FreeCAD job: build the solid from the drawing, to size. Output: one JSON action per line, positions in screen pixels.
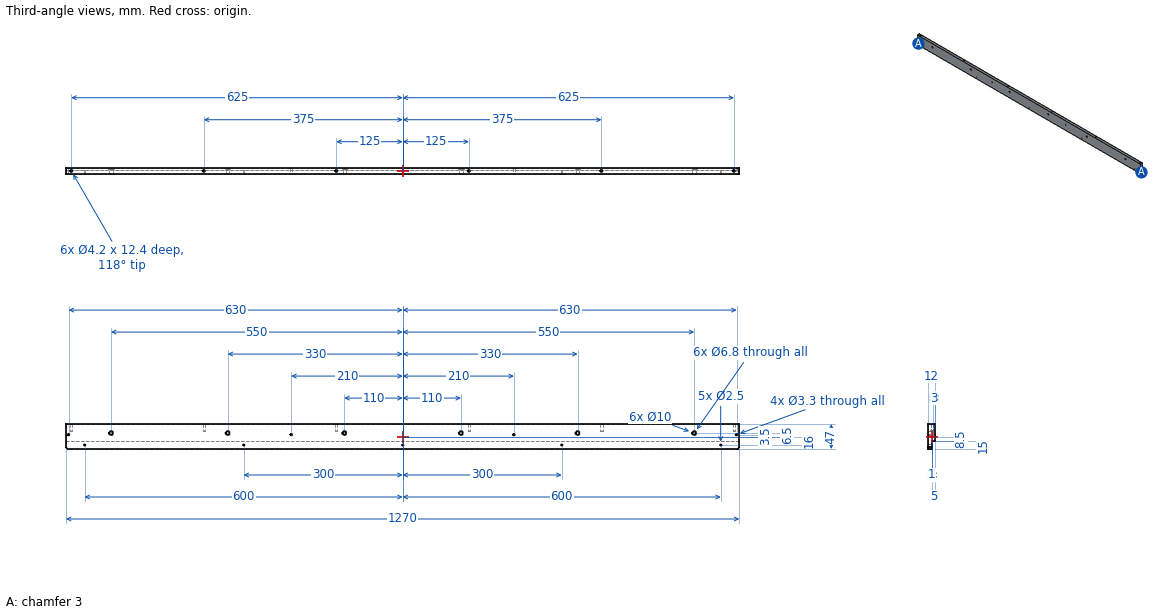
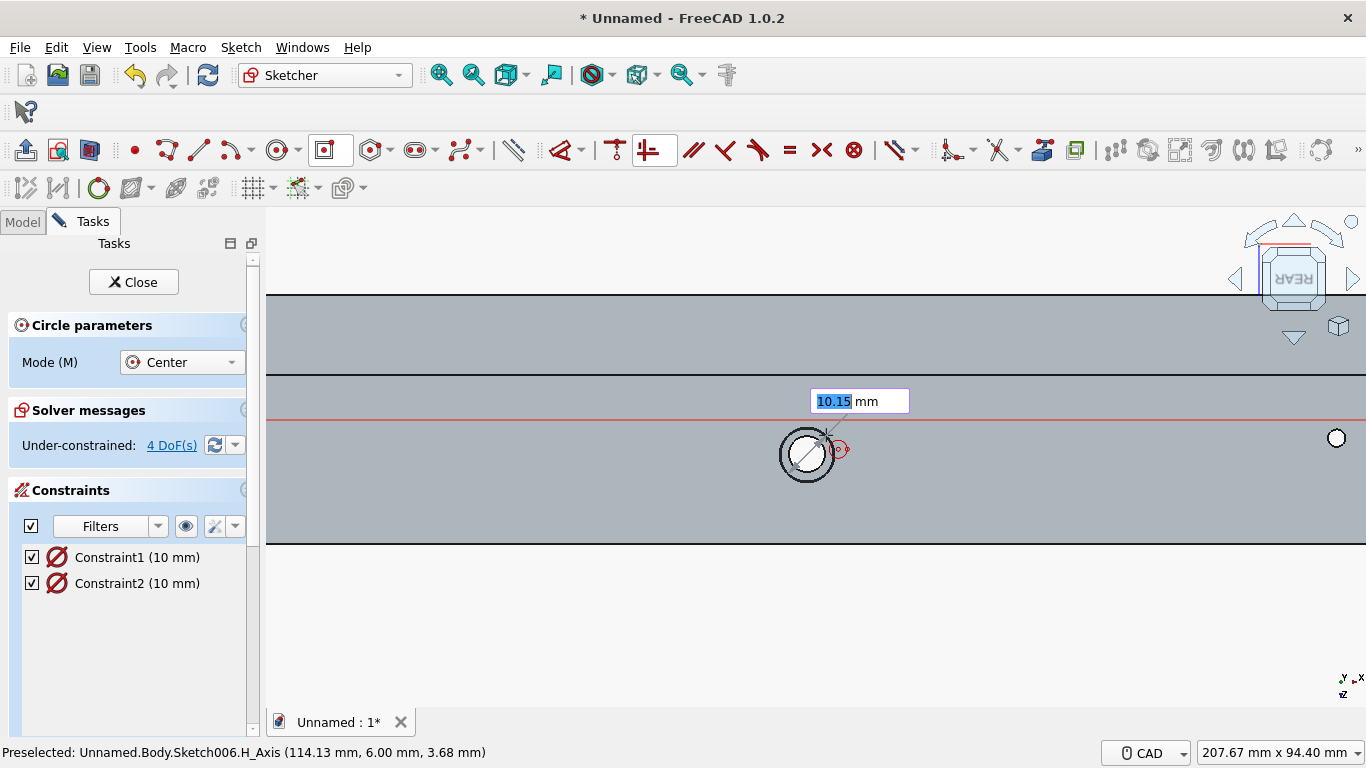
{"action": "type", "text": "10"}
{"action": "key", "text": "Return"}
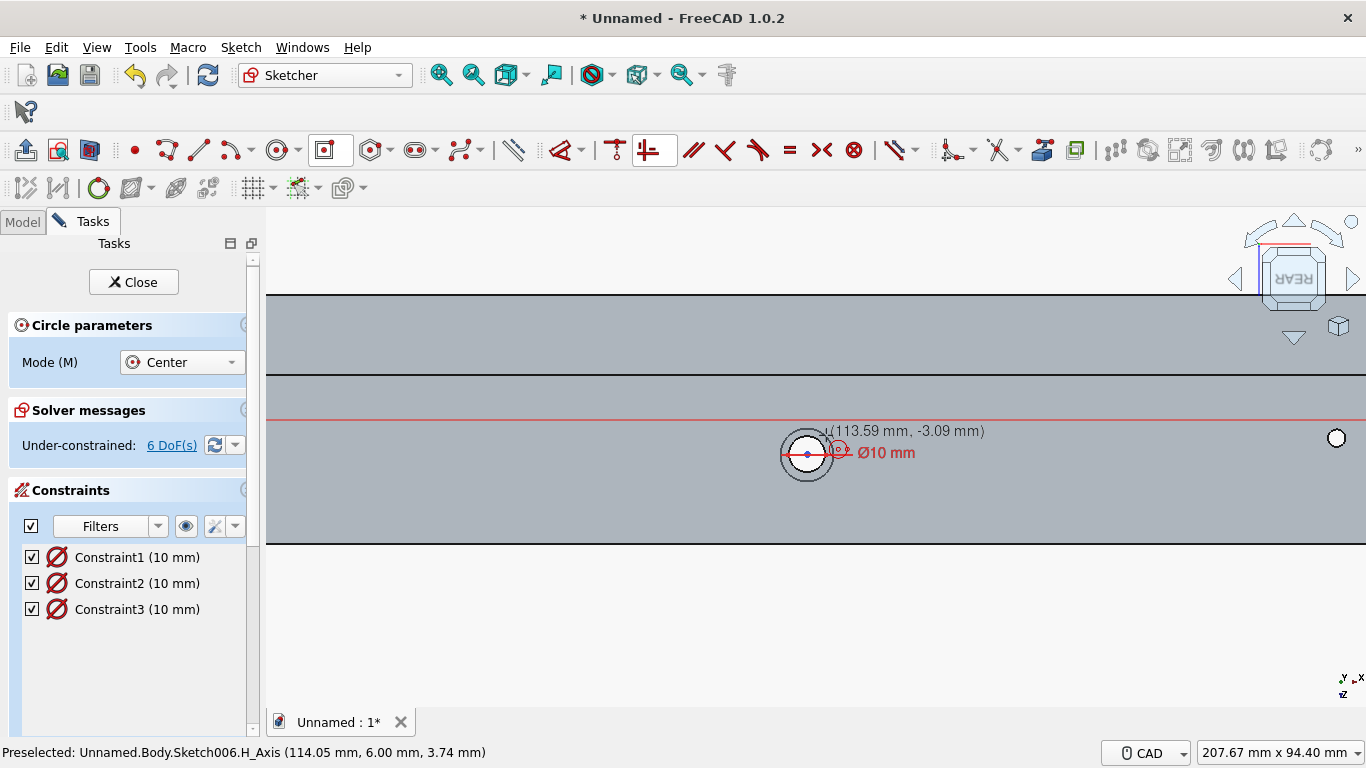
{"action": "scroll", "coordinate": [813, 458], "scroll_direction": "down", "scroll_amount": 11}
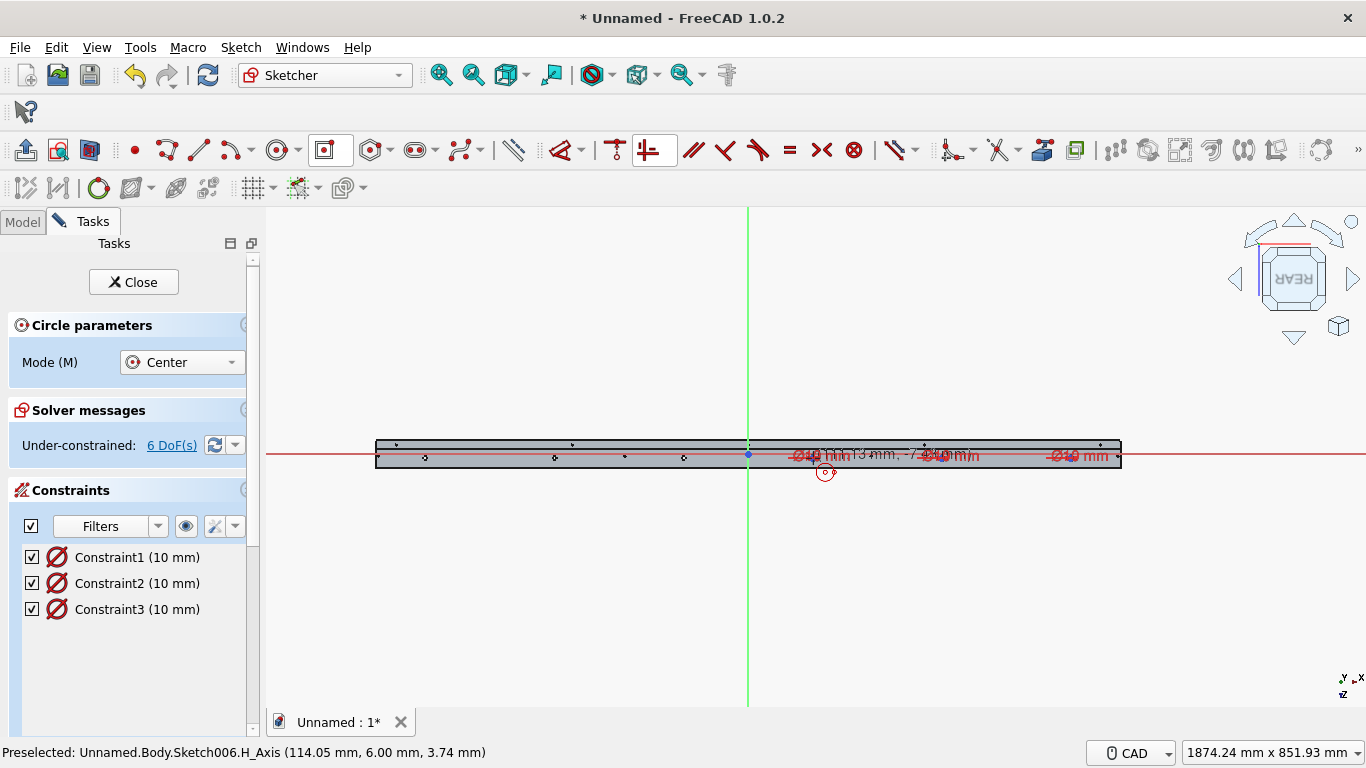
{"action": "scroll", "coordinate": [684, 458], "scroll_direction": "up", "scroll_amount": 11}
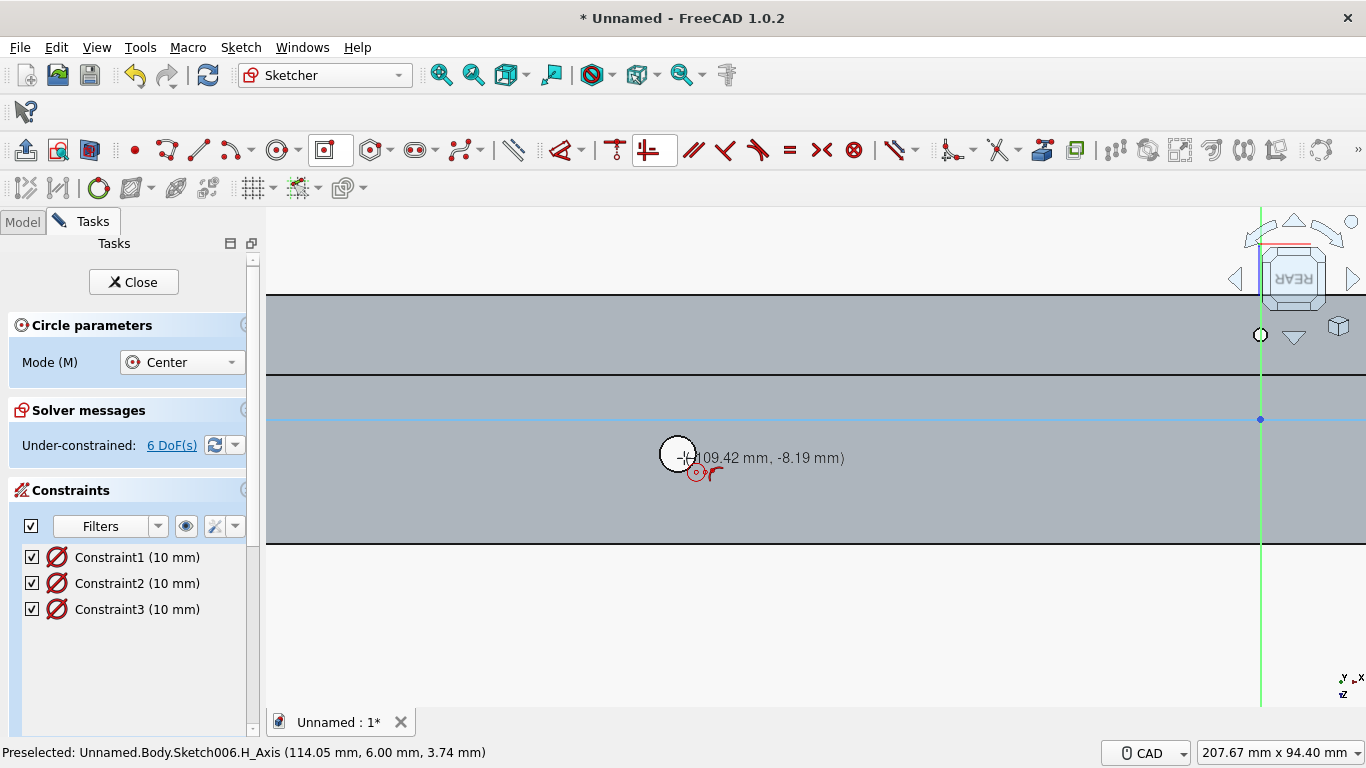
{"action": "left_click", "coordinate": [678, 454]}
{"action": "mouse_move", "coordinate": [697, 435]}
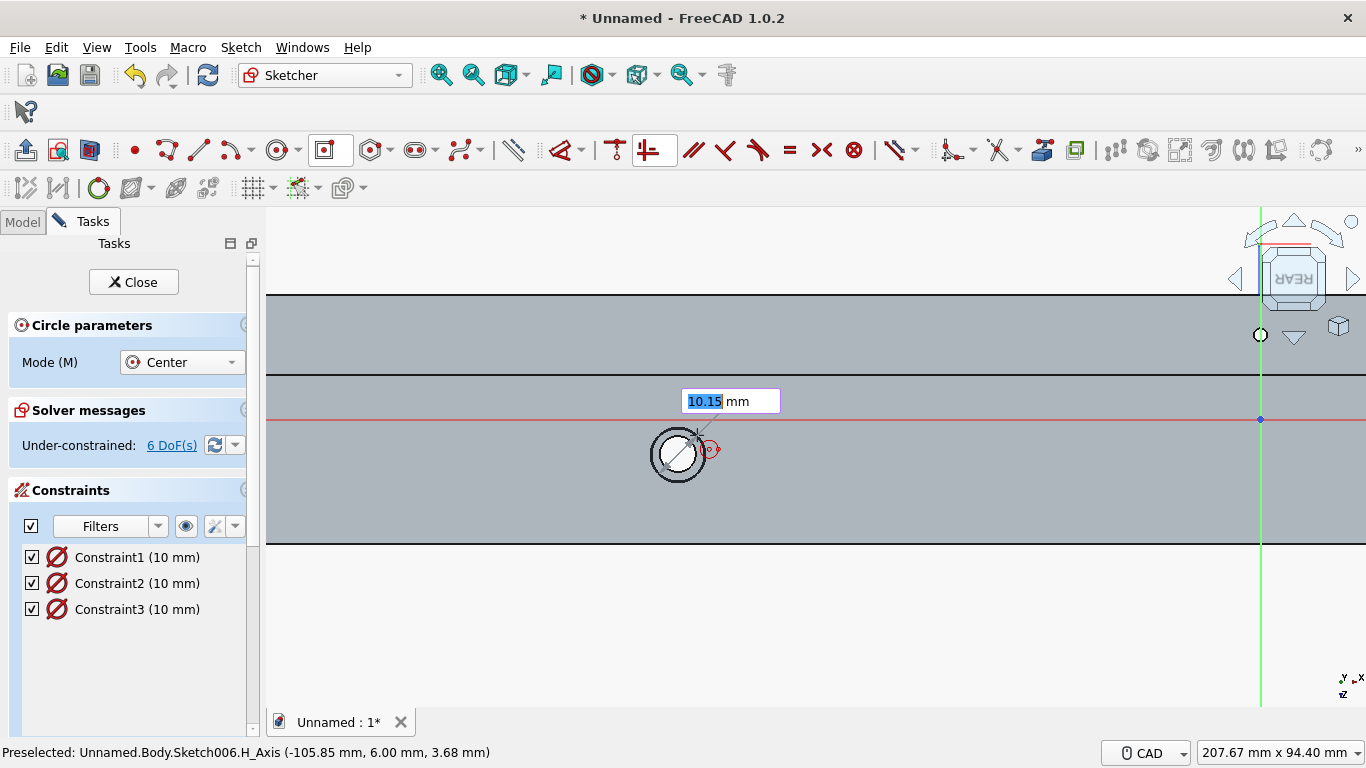
{"action": "type", "text": "10"}
{"action": "key", "text": "Return"}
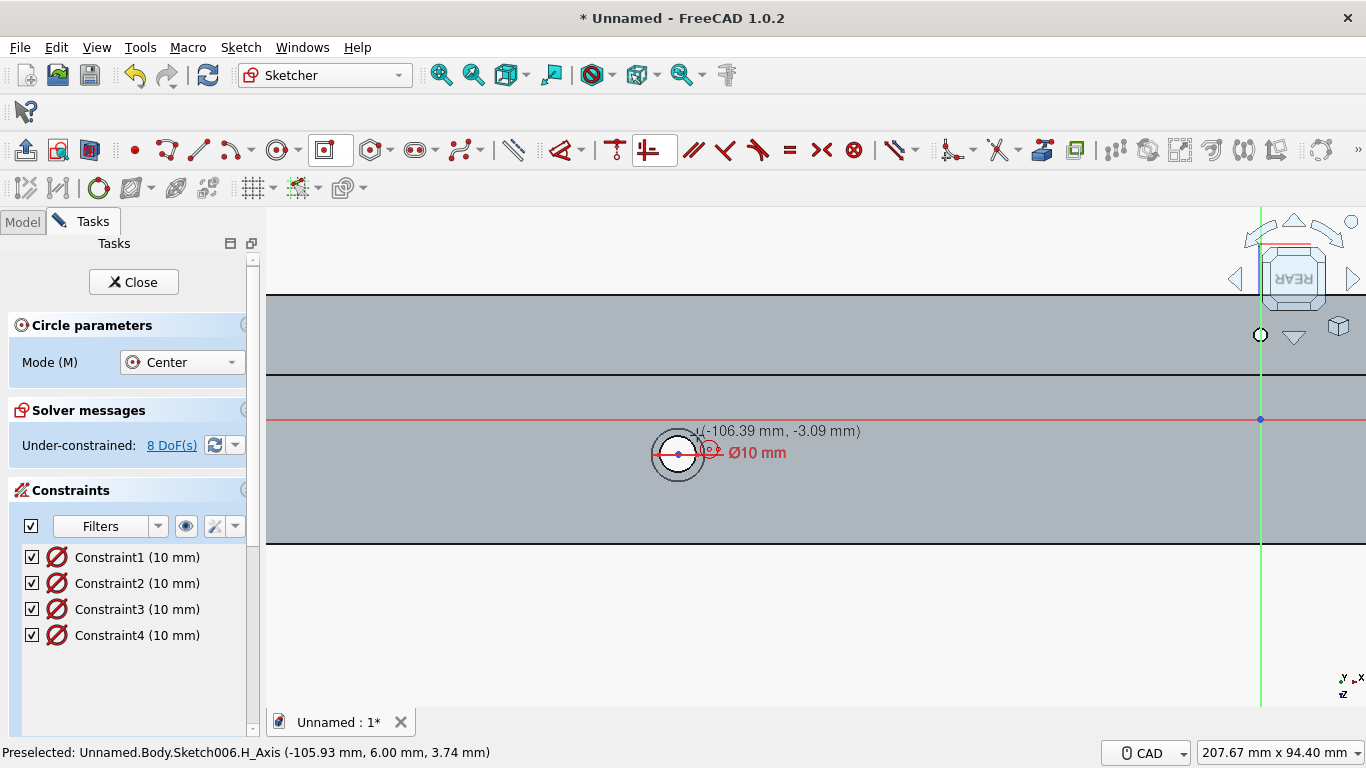
{"action": "scroll", "coordinate": [684, 458], "scroll_direction": "down", "scroll_amount": 11}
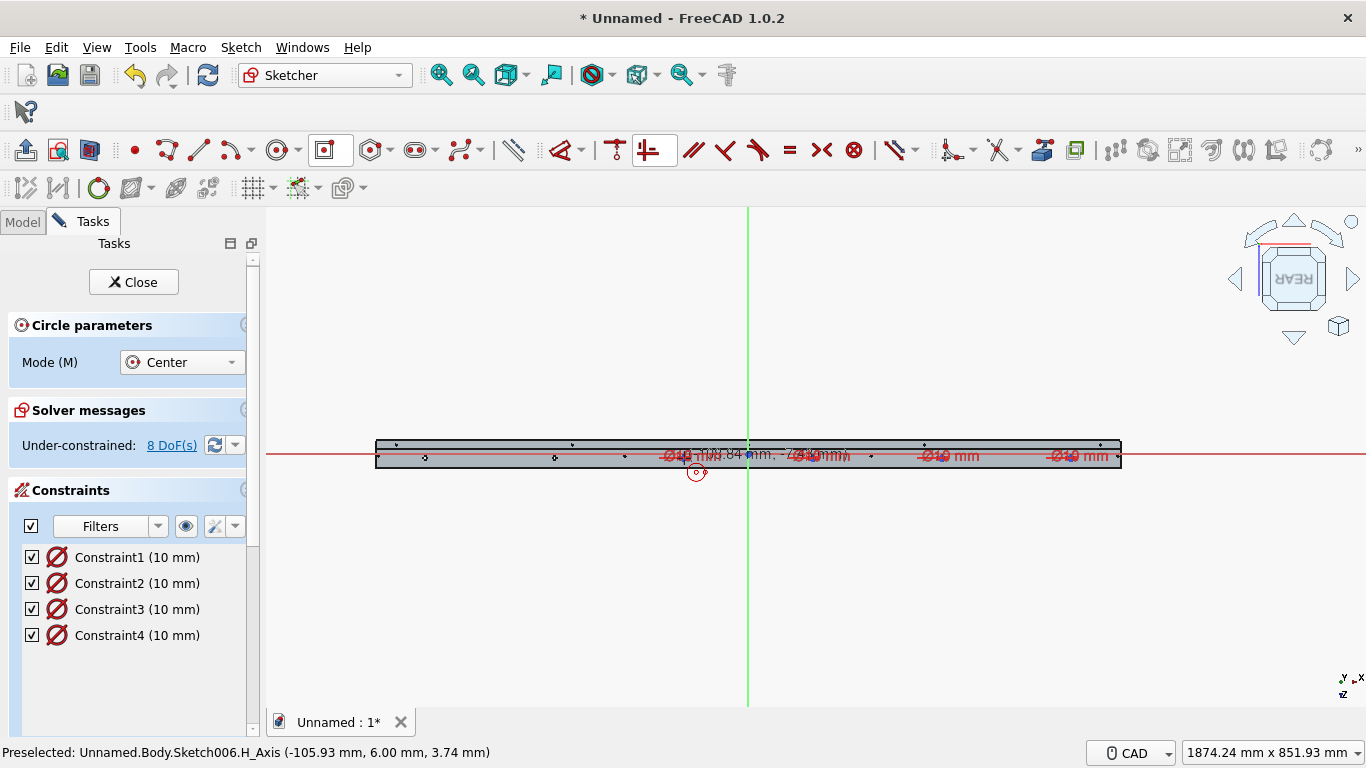
{"action": "scroll", "coordinate": [555, 458], "scroll_direction": "up", "scroll_amount": 11}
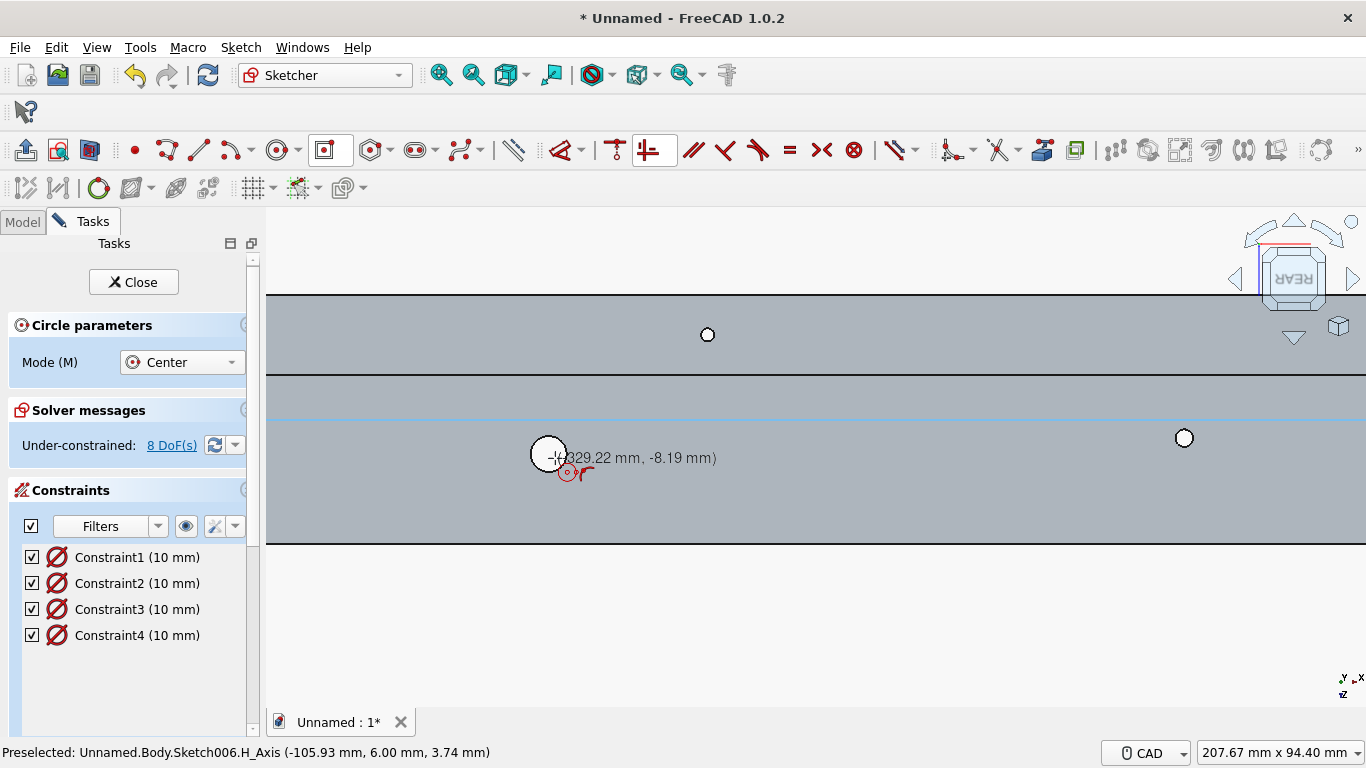
{"action": "left_click", "coordinate": [549, 454]}
{"action": "mouse_move", "coordinate": [567, 435]}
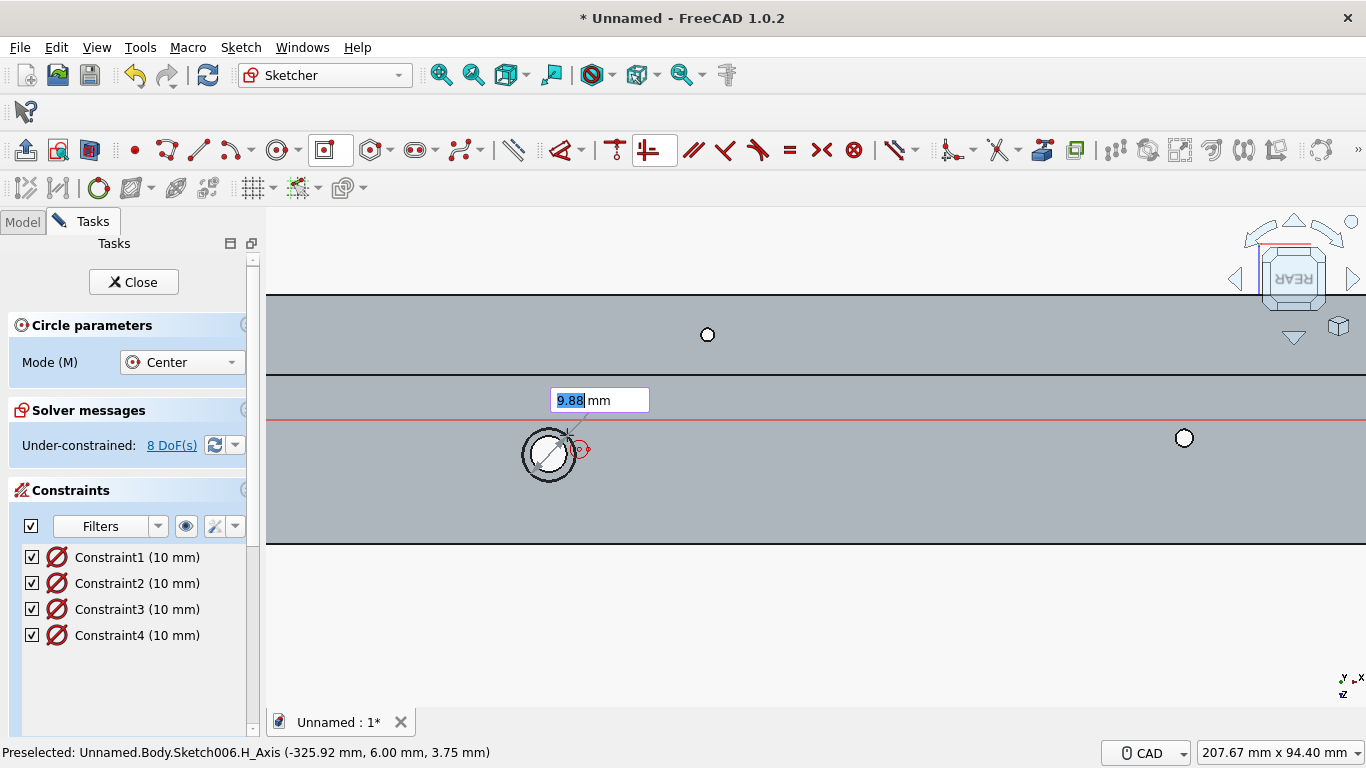
{"action": "type", "text": "10"}
{"action": "key", "text": "Return"}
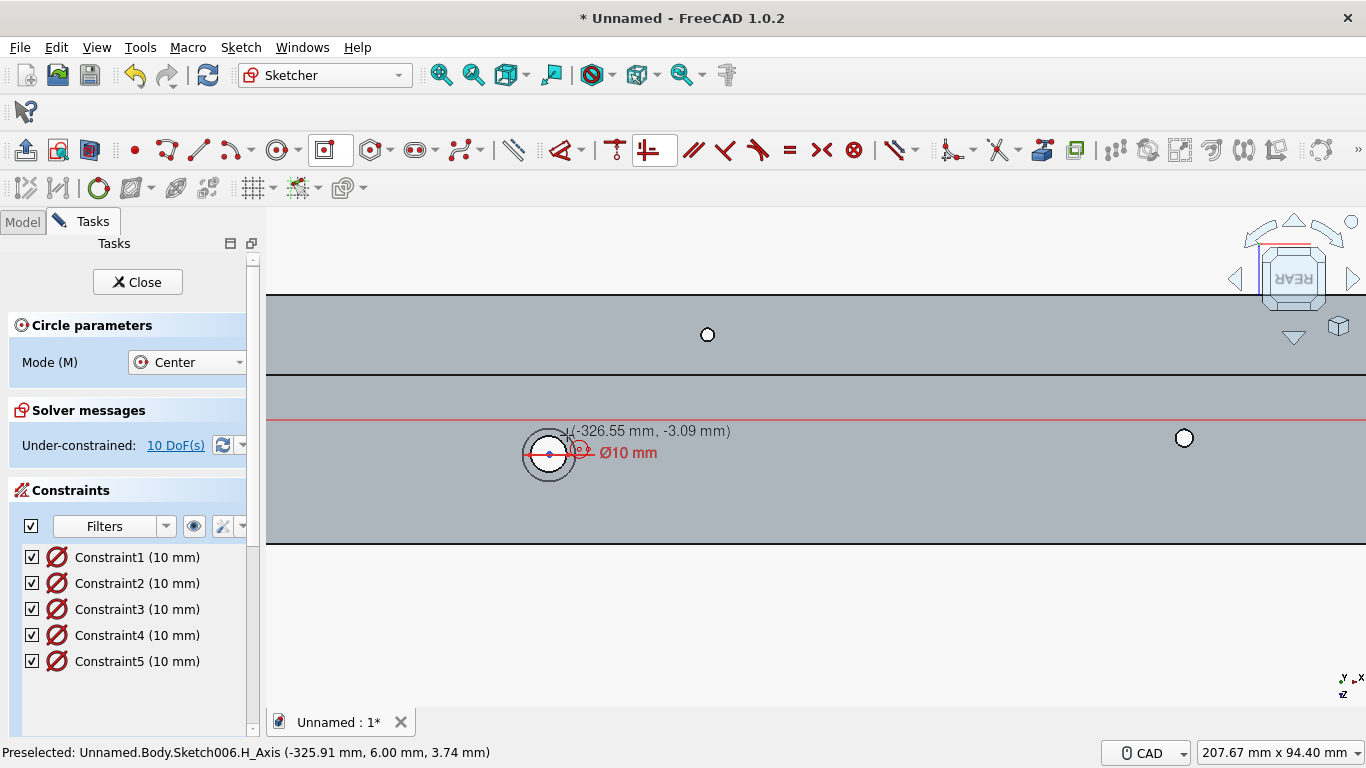
{"action": "scroll", "coordinate": [554, 458], "scroll_direction": "down", "scroll_amount": 11}